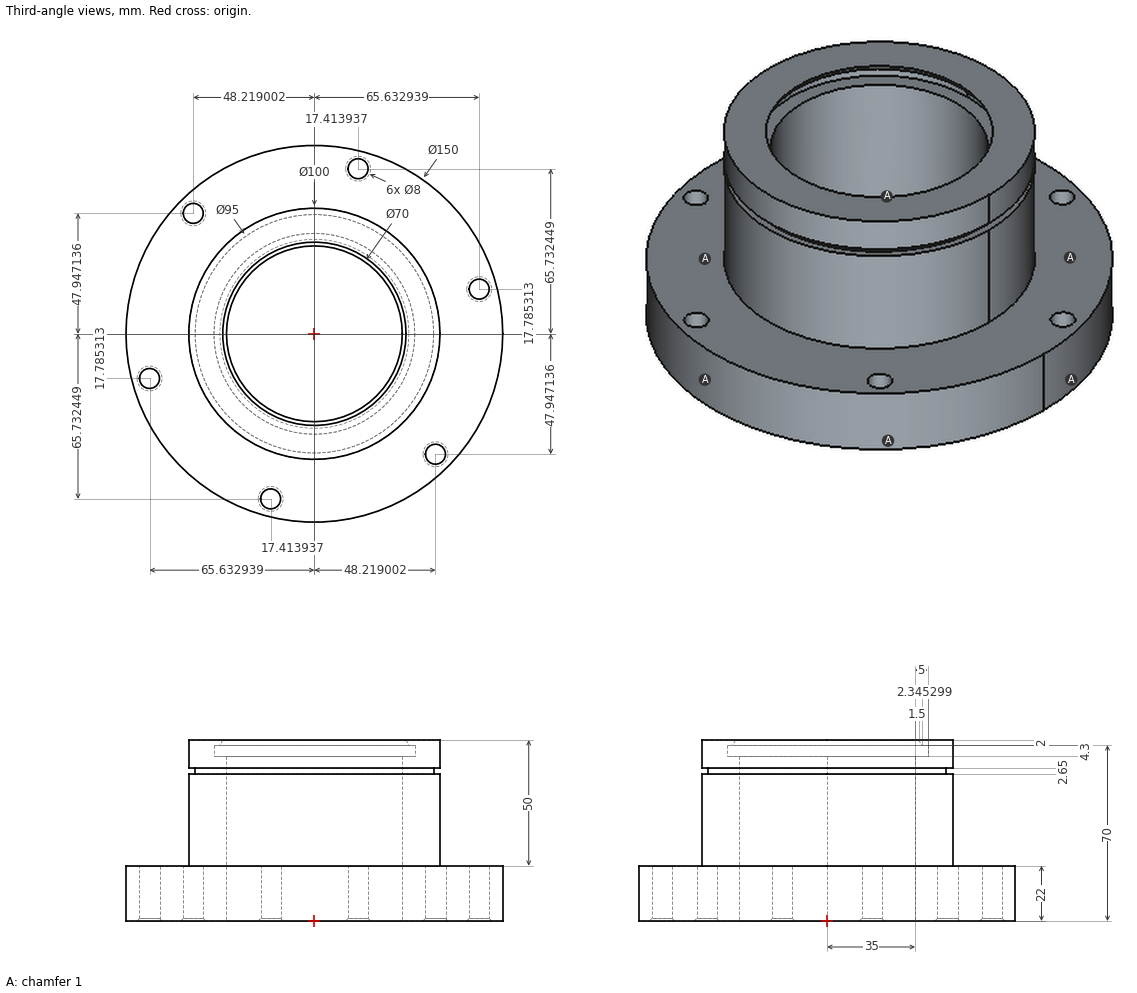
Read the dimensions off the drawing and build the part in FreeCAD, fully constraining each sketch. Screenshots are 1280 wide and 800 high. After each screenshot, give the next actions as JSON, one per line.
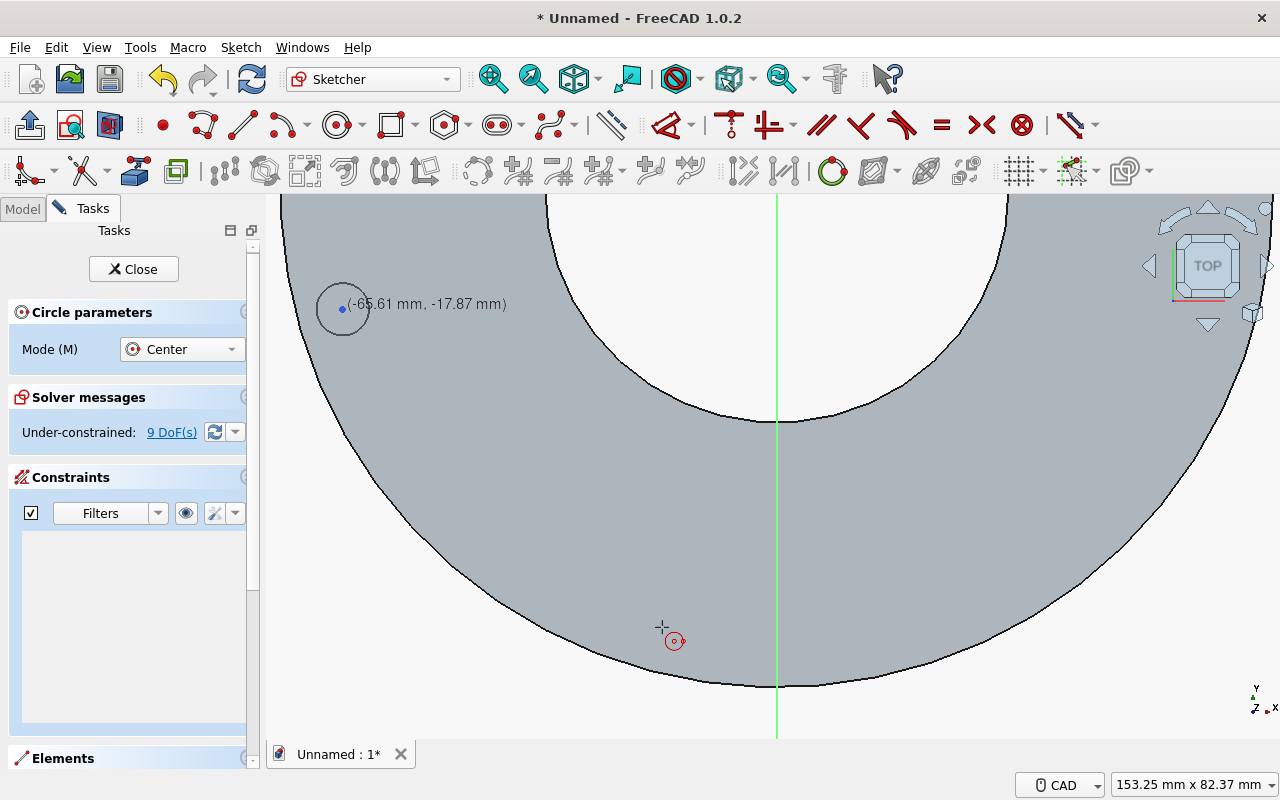
{"action": "left_click", "coordinate": [662, 626]}
{"action": "left_click", "coordinate": [680, 607]}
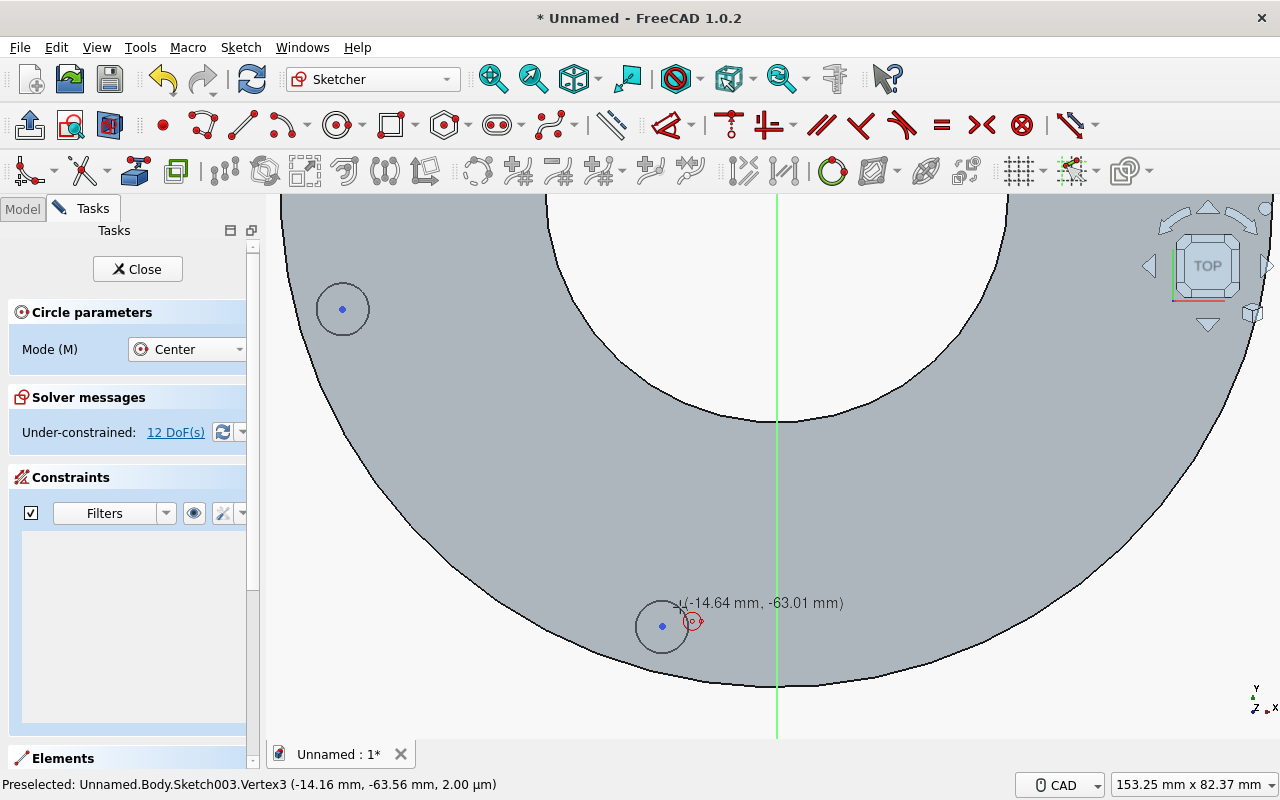
{"action": "left_click", "coordinate": [1096, 508]}
{"action": "left_click", "coordinate": [1115, 490]}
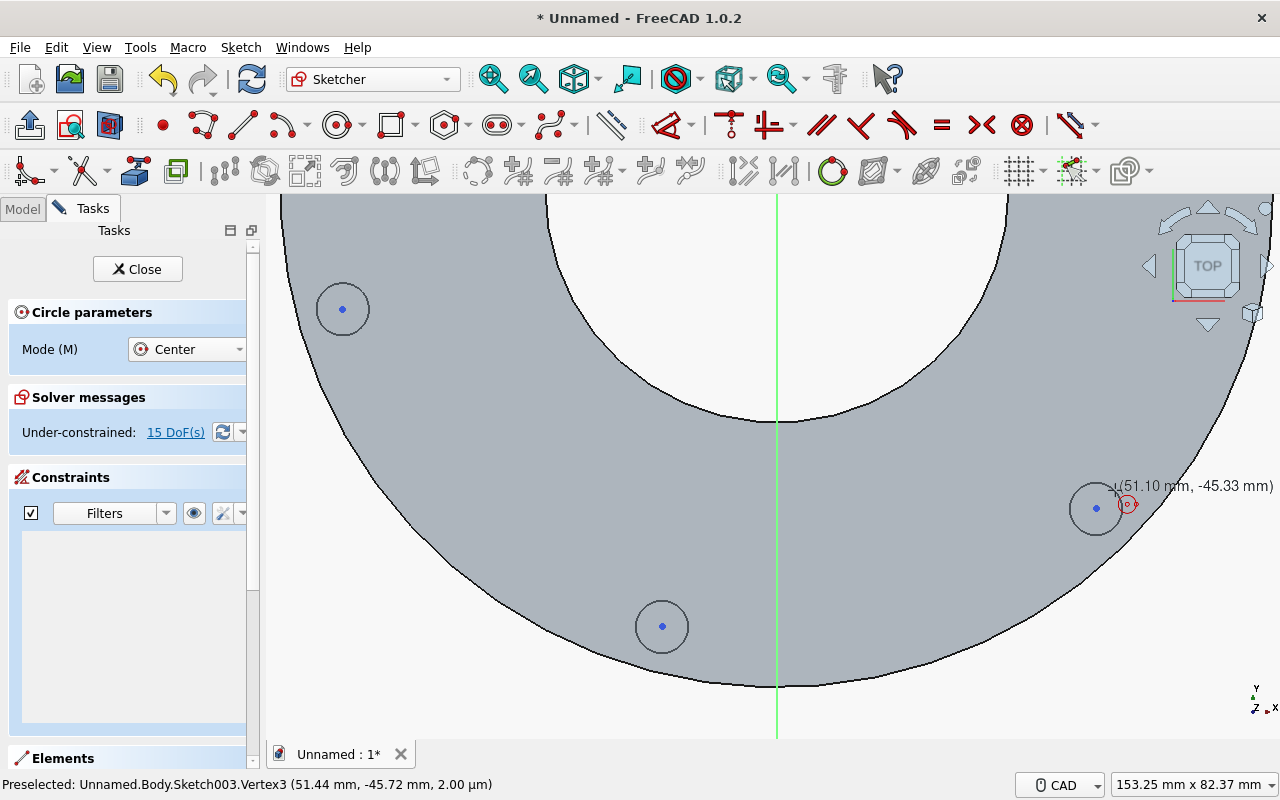
{"action": "scroll", "coordinate": [662, 627], "scroll_direction": "down", "scroll_amount": 5}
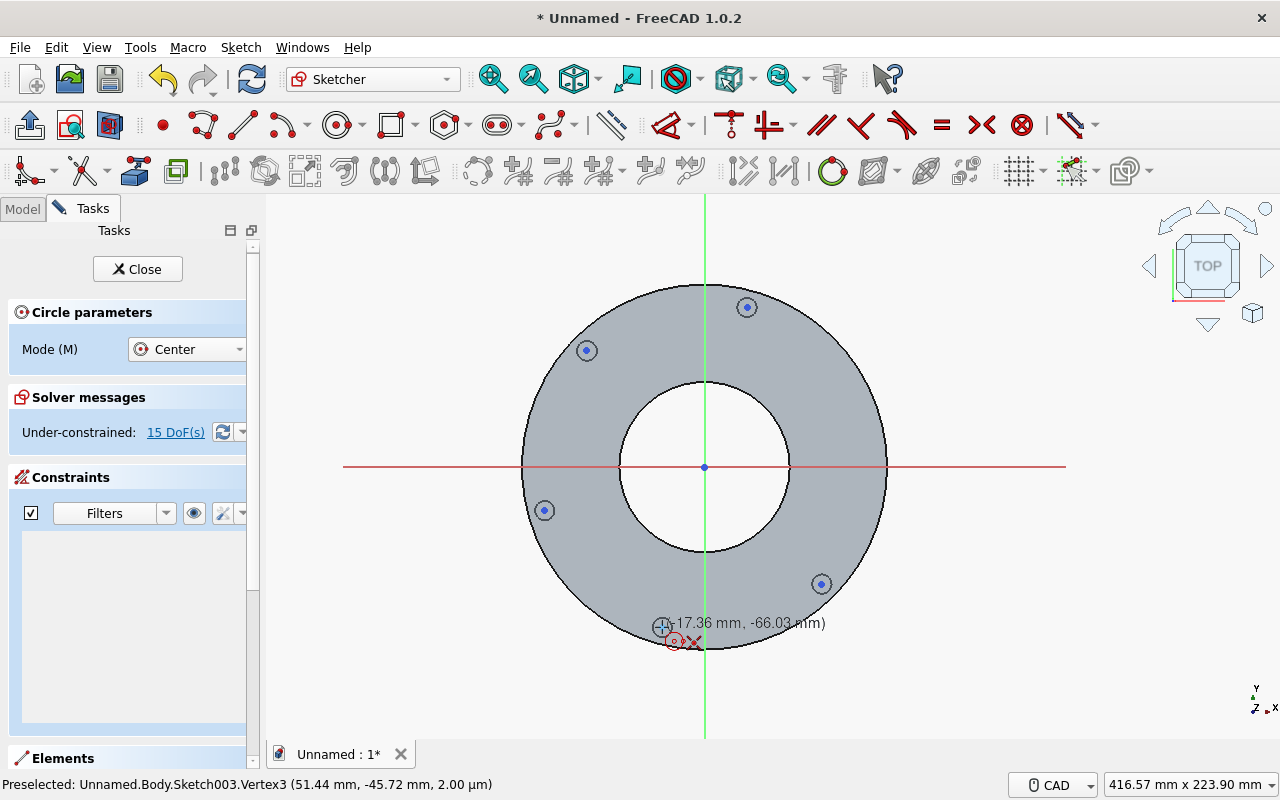
{"action": "scroll", "coordinate": [864, 424], "scroll_direction": "up", "scroll_amount": 5}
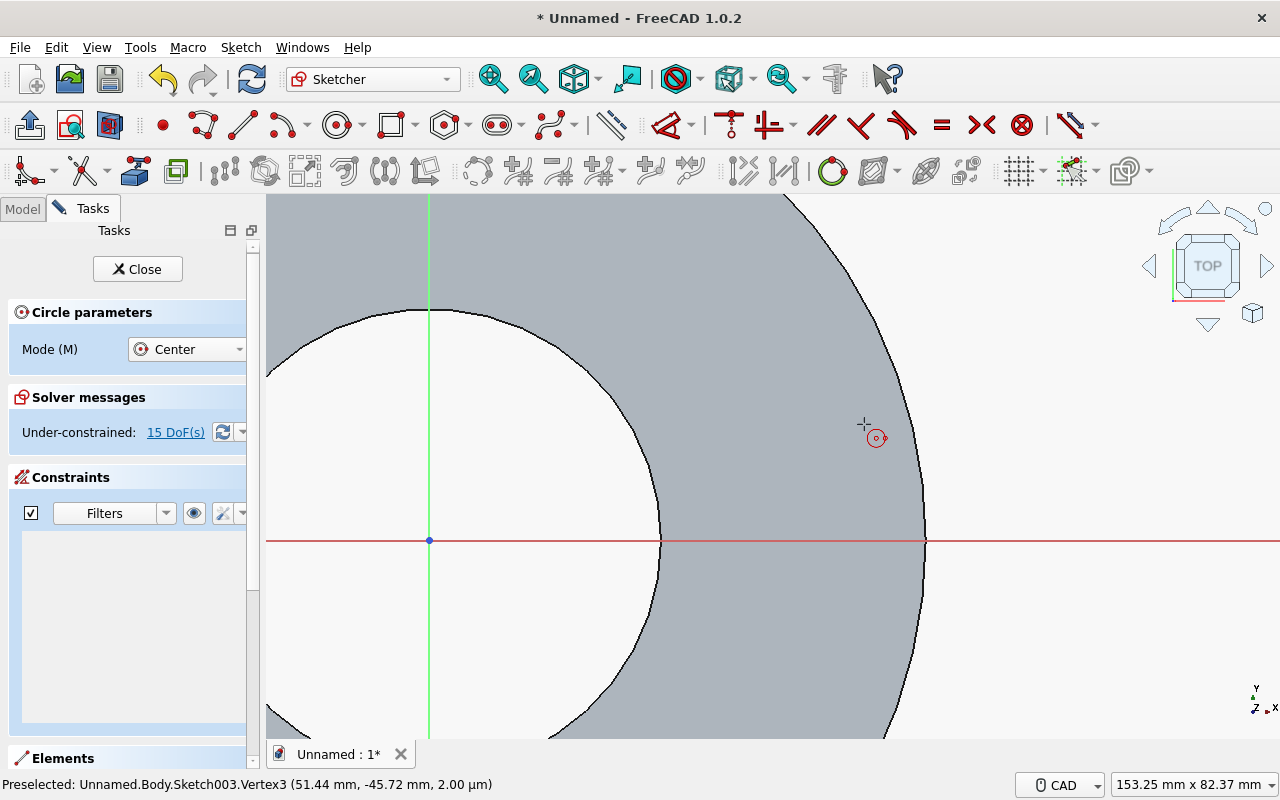
{"action": "left_click", "coordinate": [864, 423]}
{"action": "left_click", "coordinate": [882, 404]}
{"action": "key", "text": "Escape"}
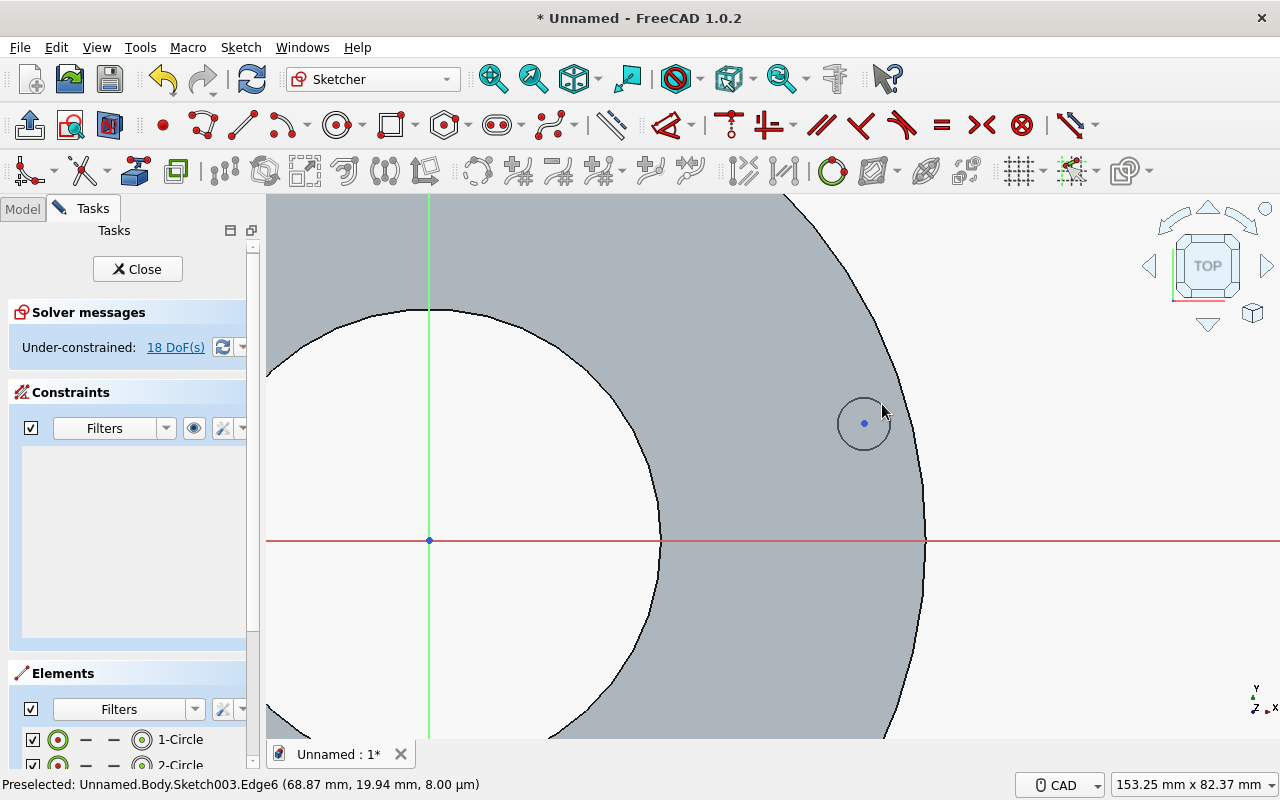
{"action": "scroll", "coordinate": [865, 423], "scroll_direction": "down", "scroll_amount": 5}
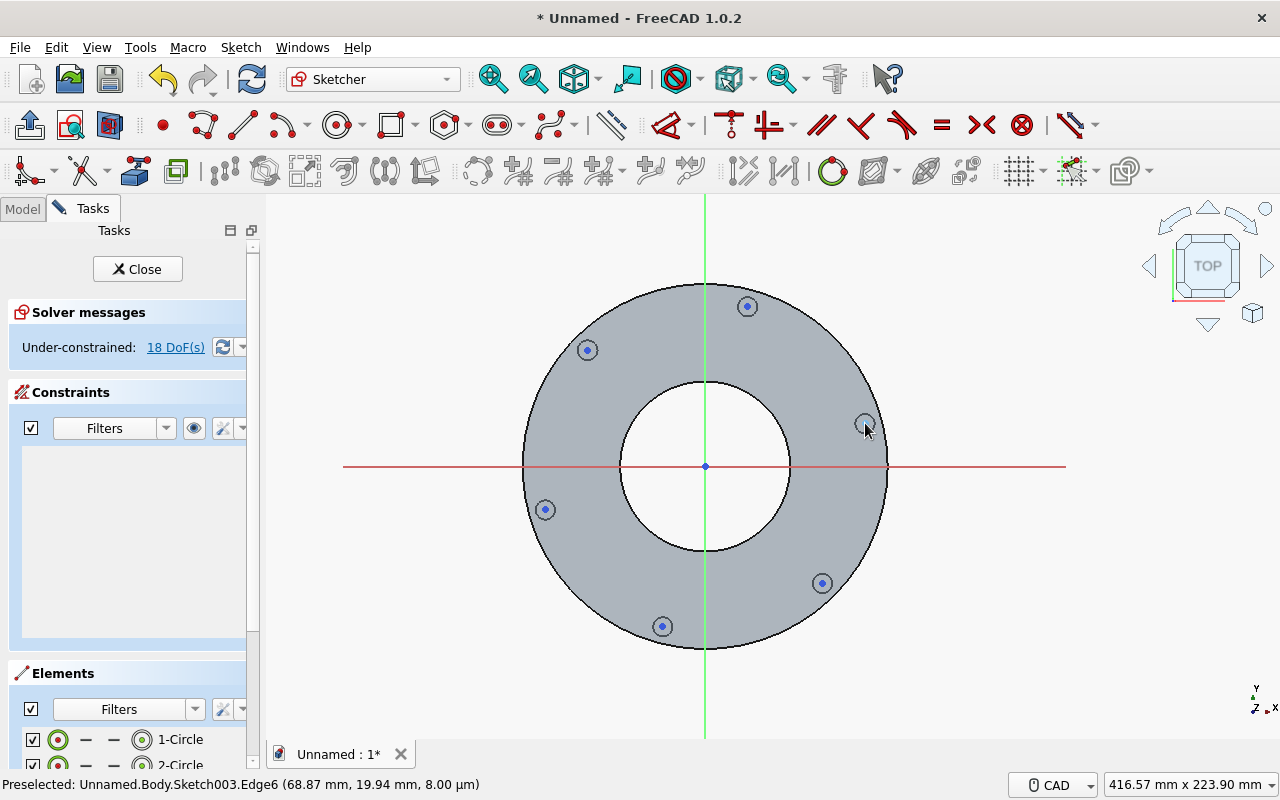
{"action": "scroll", "coordinate": [754, 300], "scroll_direction": "up", "scroll_amount": 2}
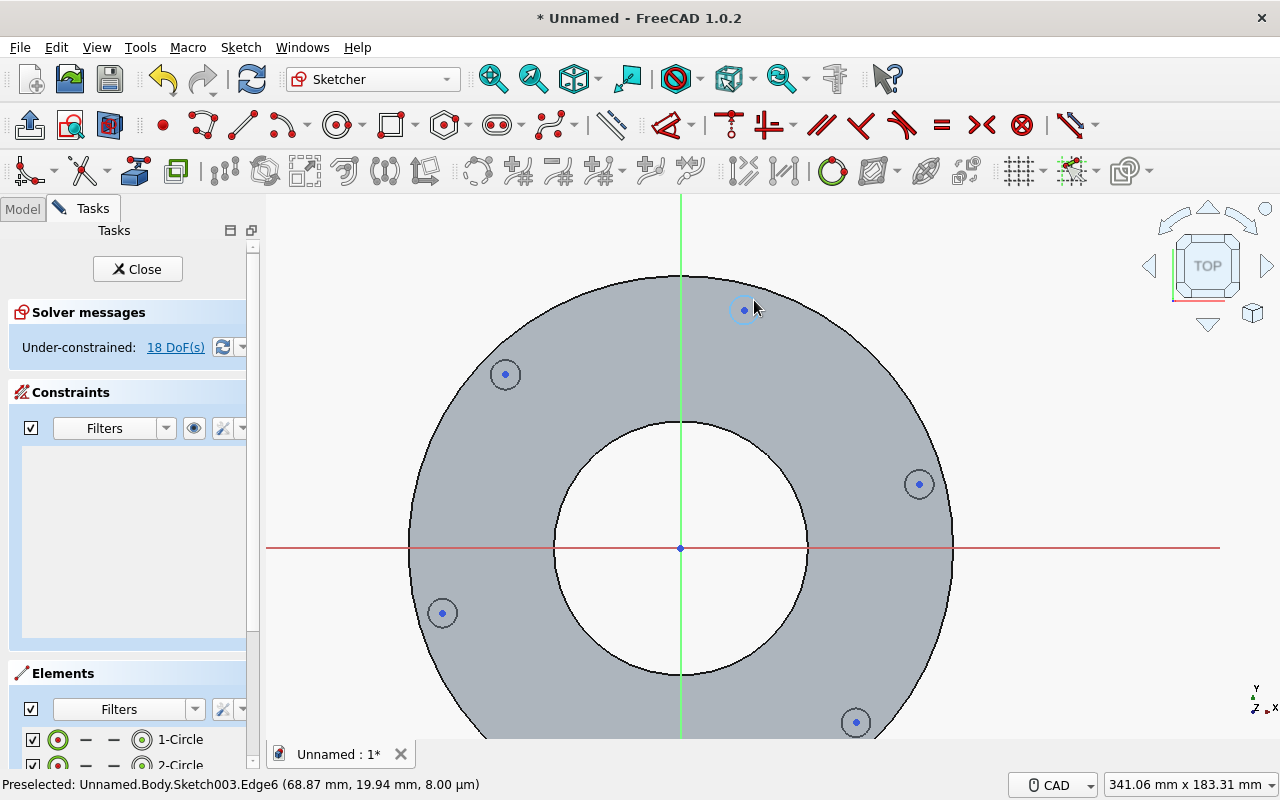
{"action": "left_click", "coordinate": [754, 300]}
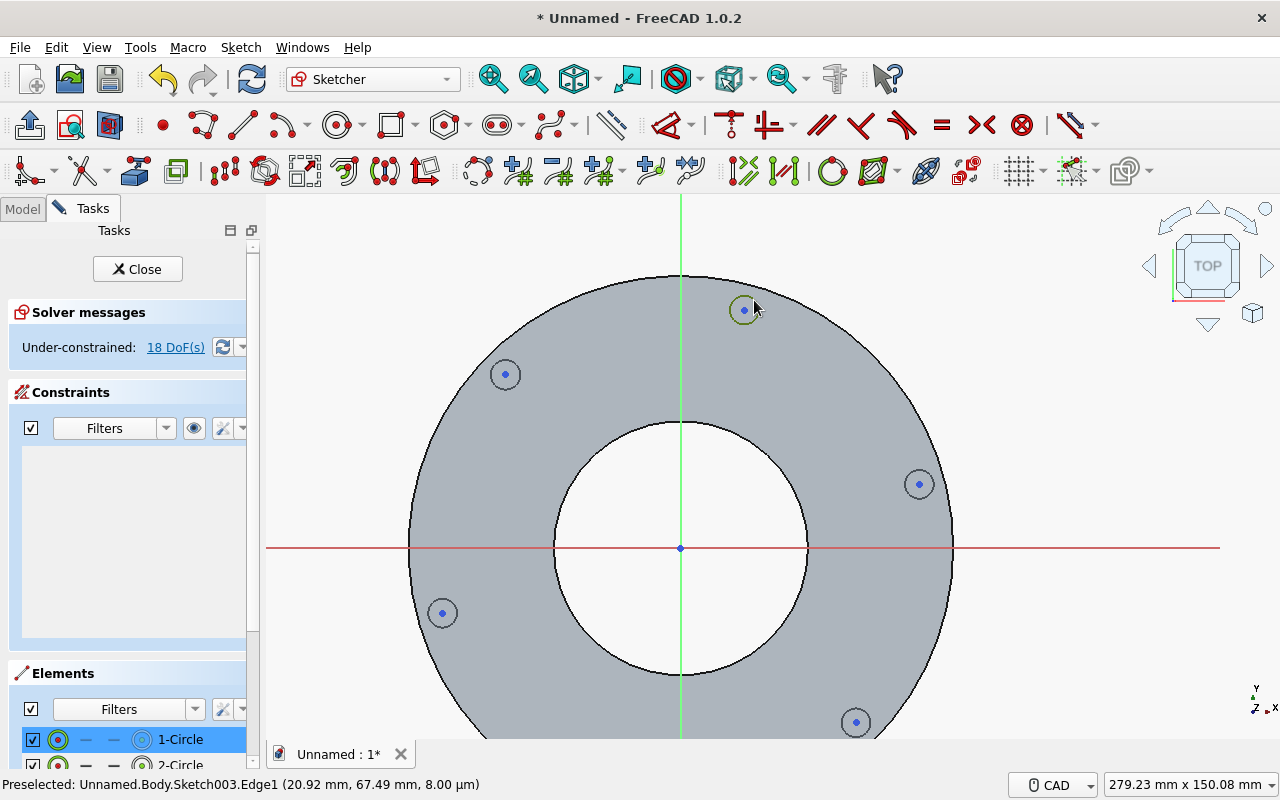
{"action": "left_click", "coordinate": [516, 364]}